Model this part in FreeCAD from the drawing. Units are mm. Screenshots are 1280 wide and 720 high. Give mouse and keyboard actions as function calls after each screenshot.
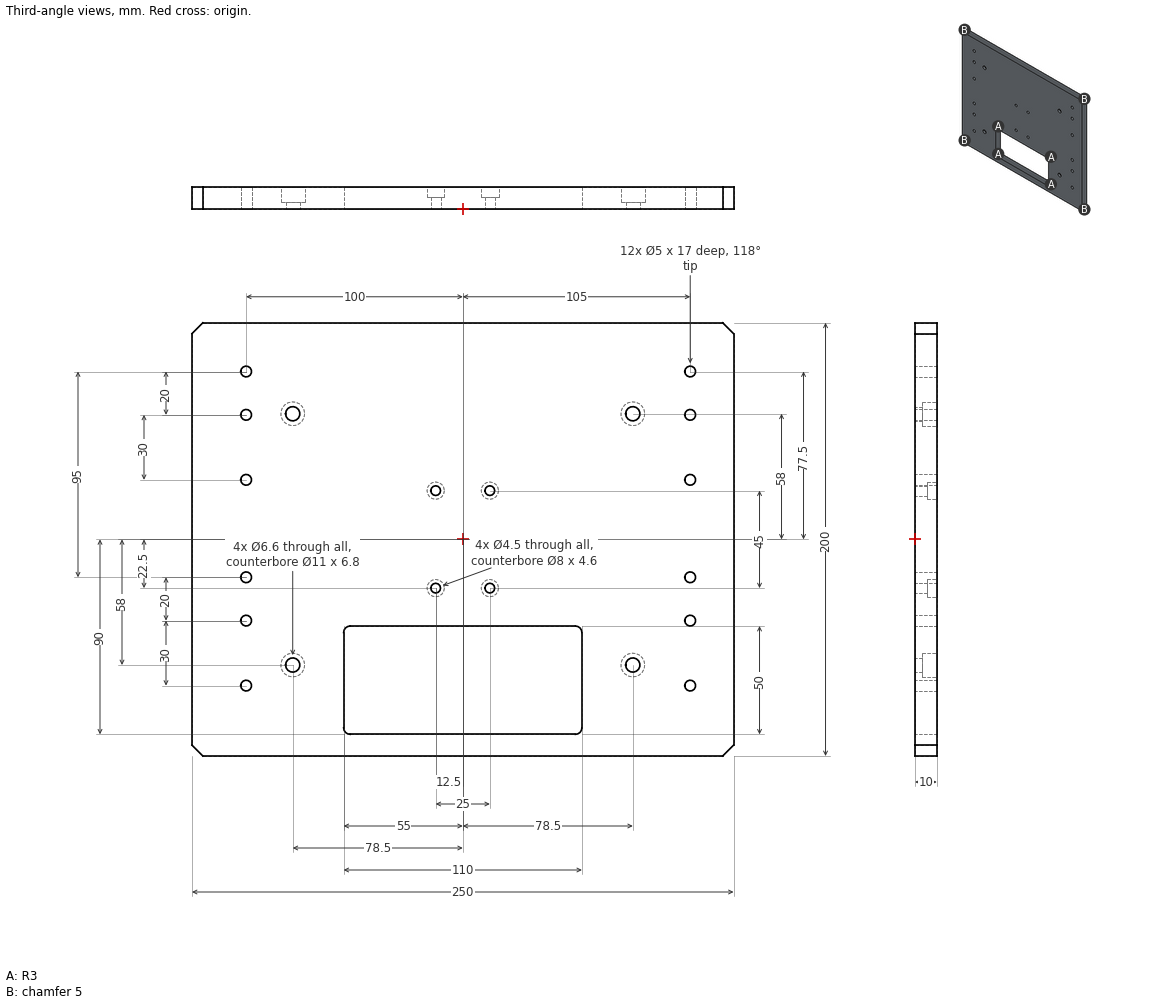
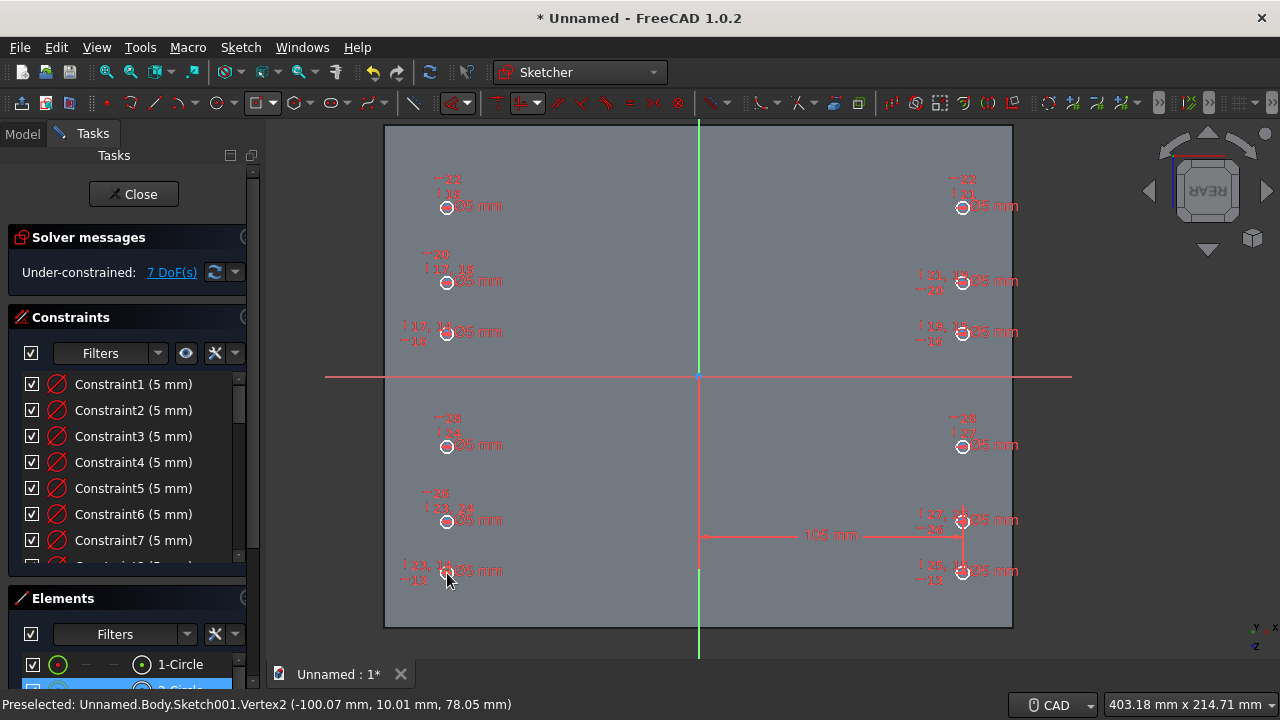
key(l)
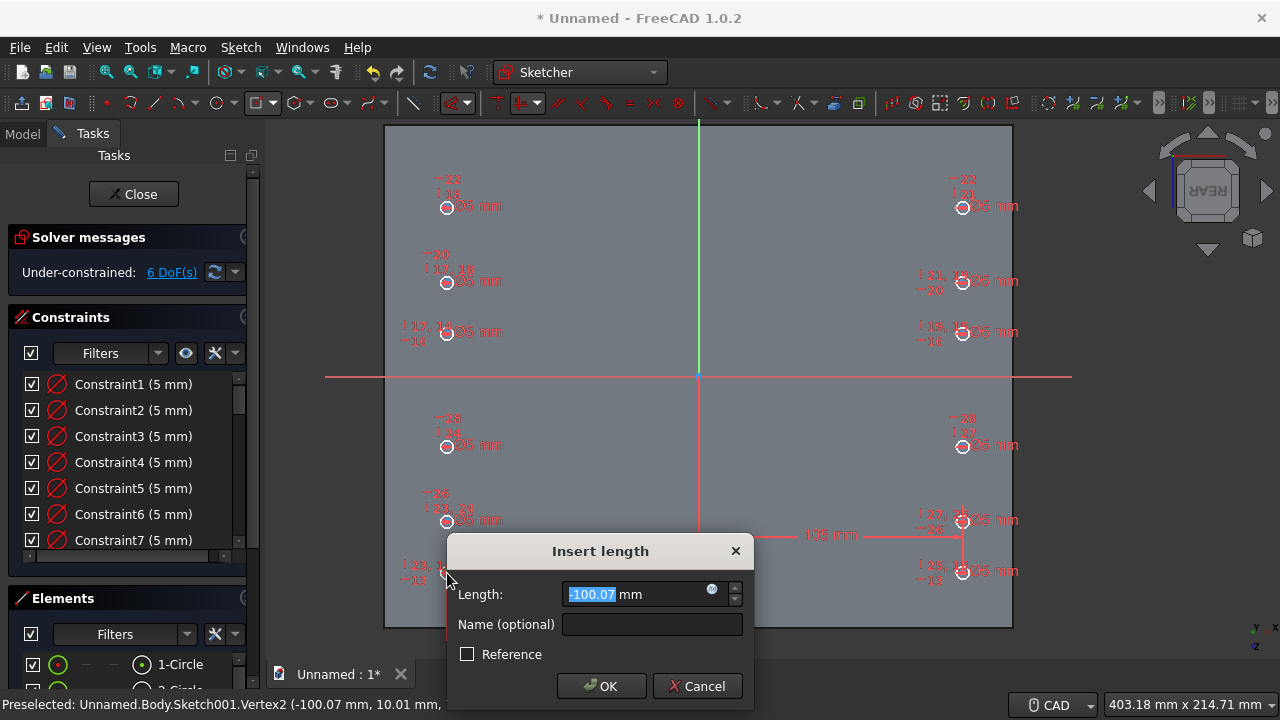
text(-100)
key(Return)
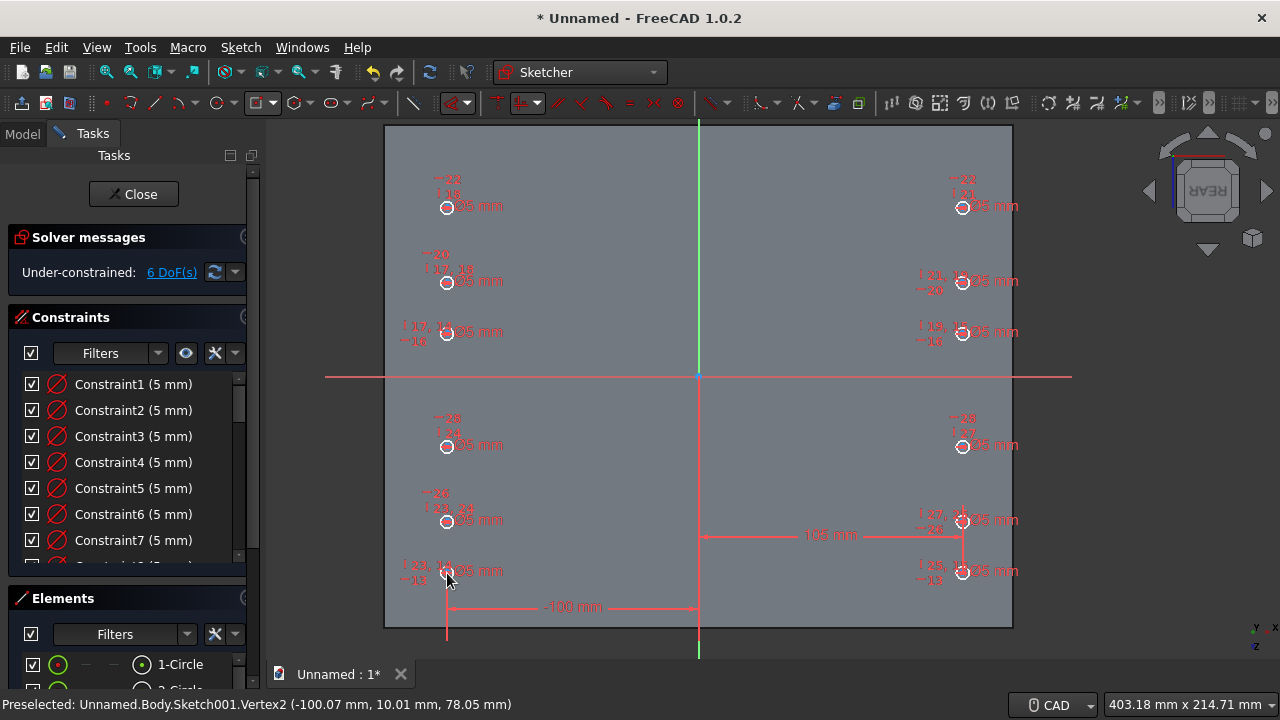
click(447, 573)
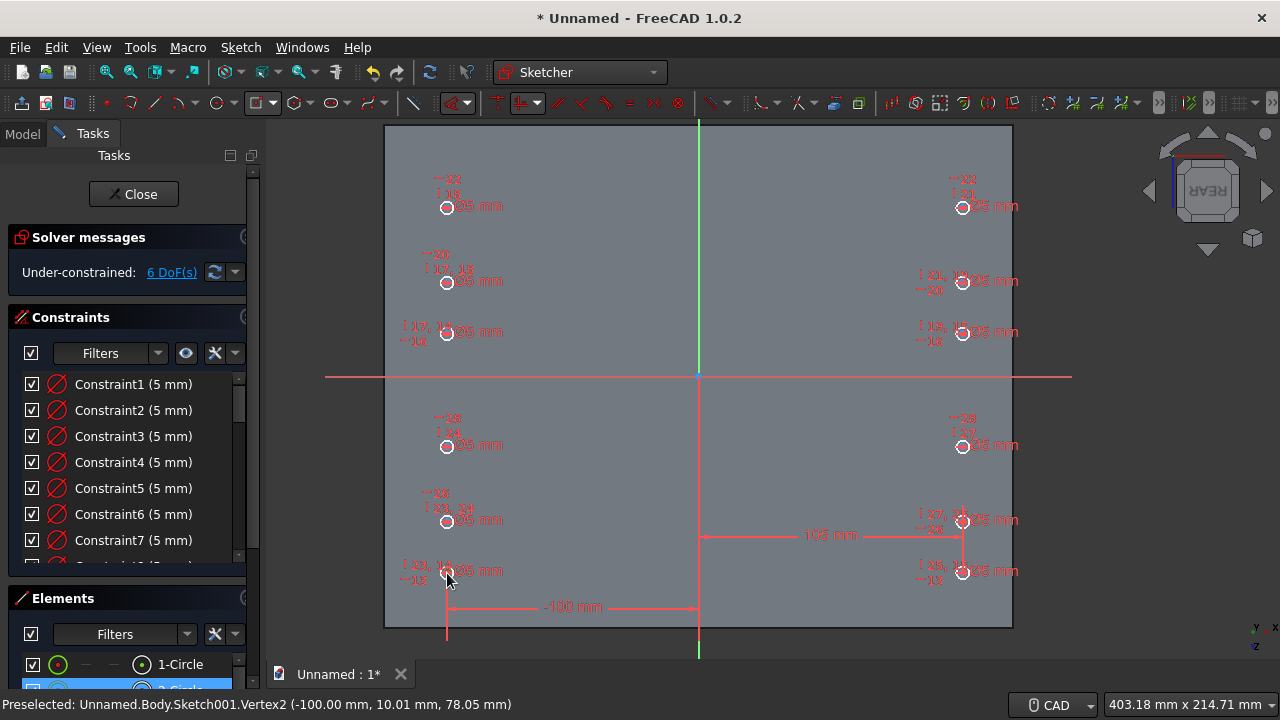
click(447, 334)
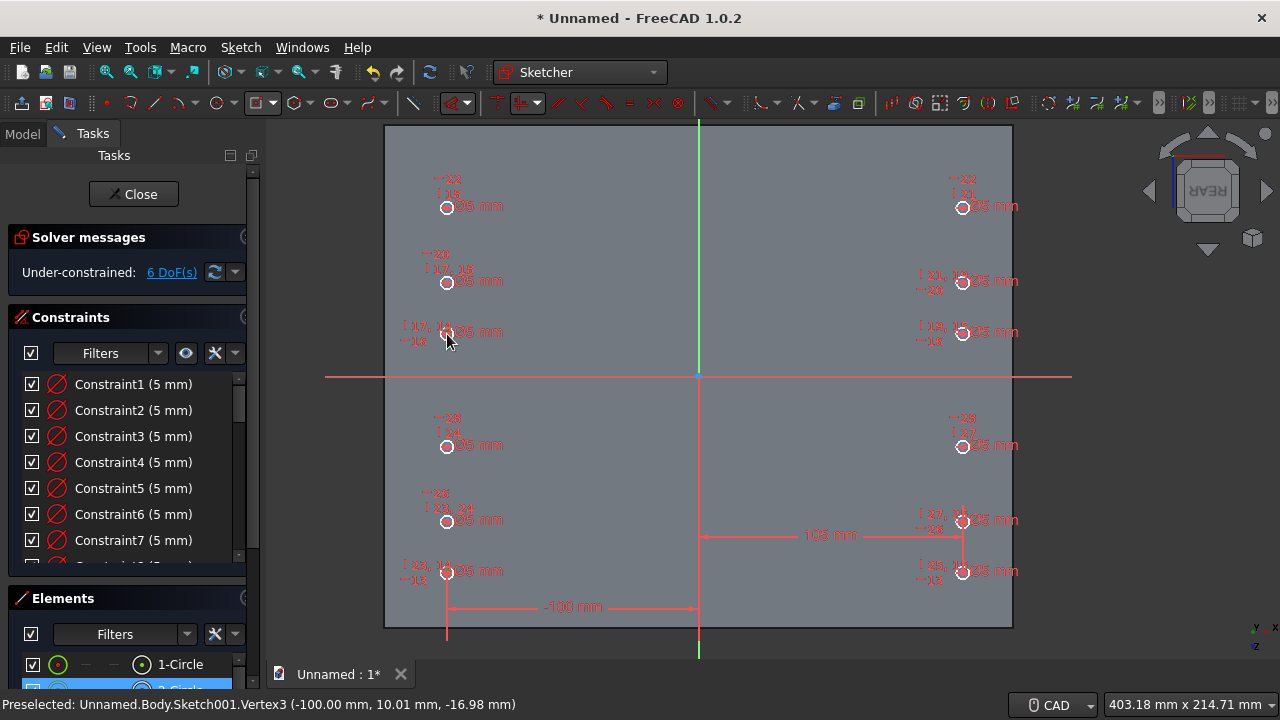
click(470, 104)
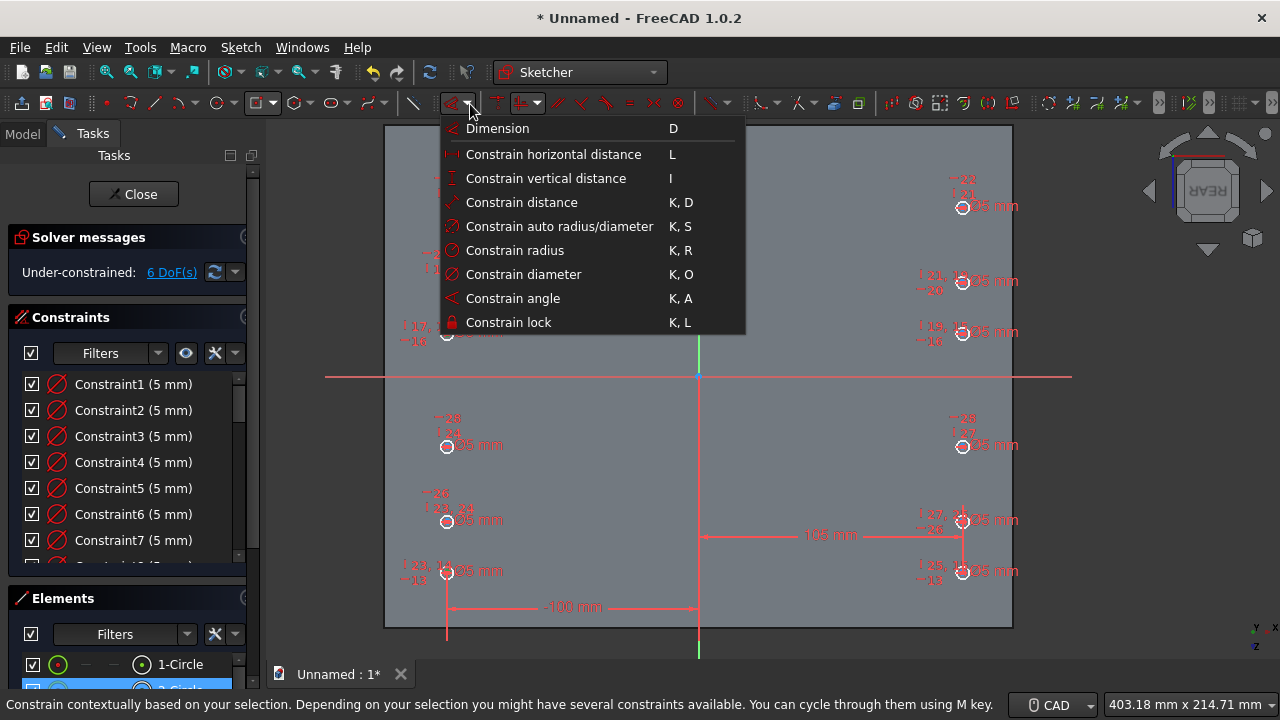
click(593, 178)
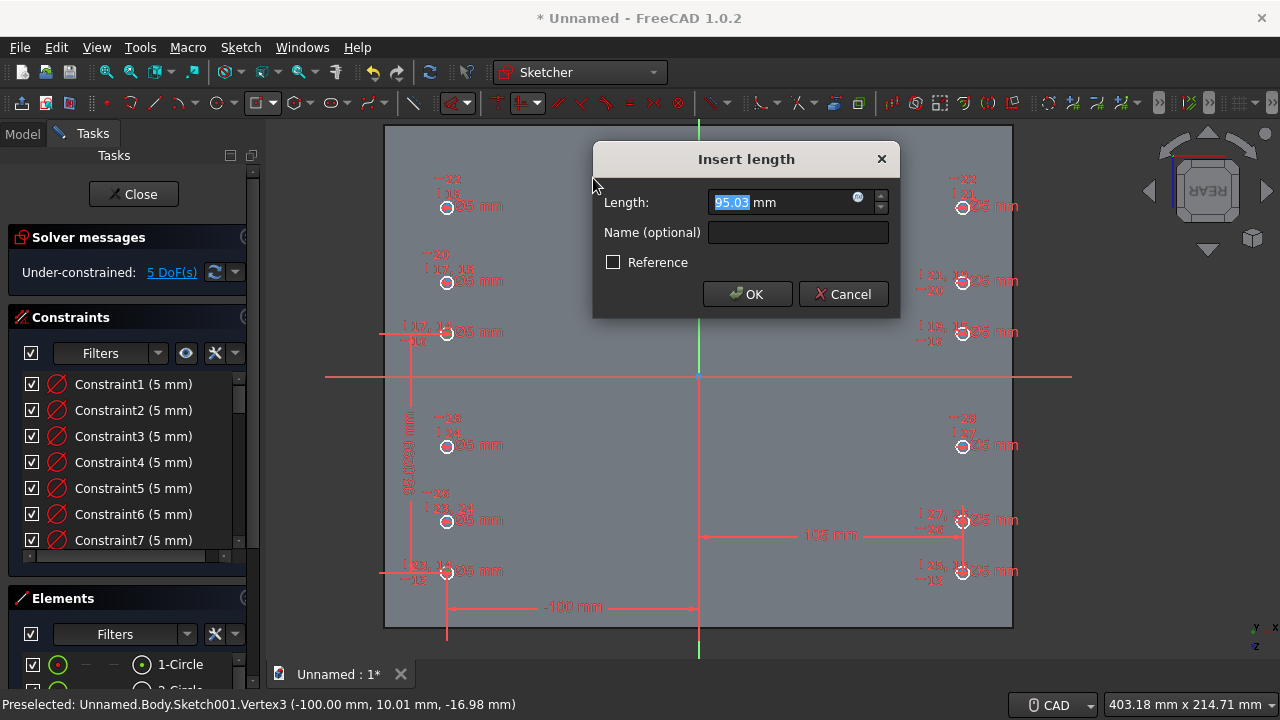
text(95)
key(Return)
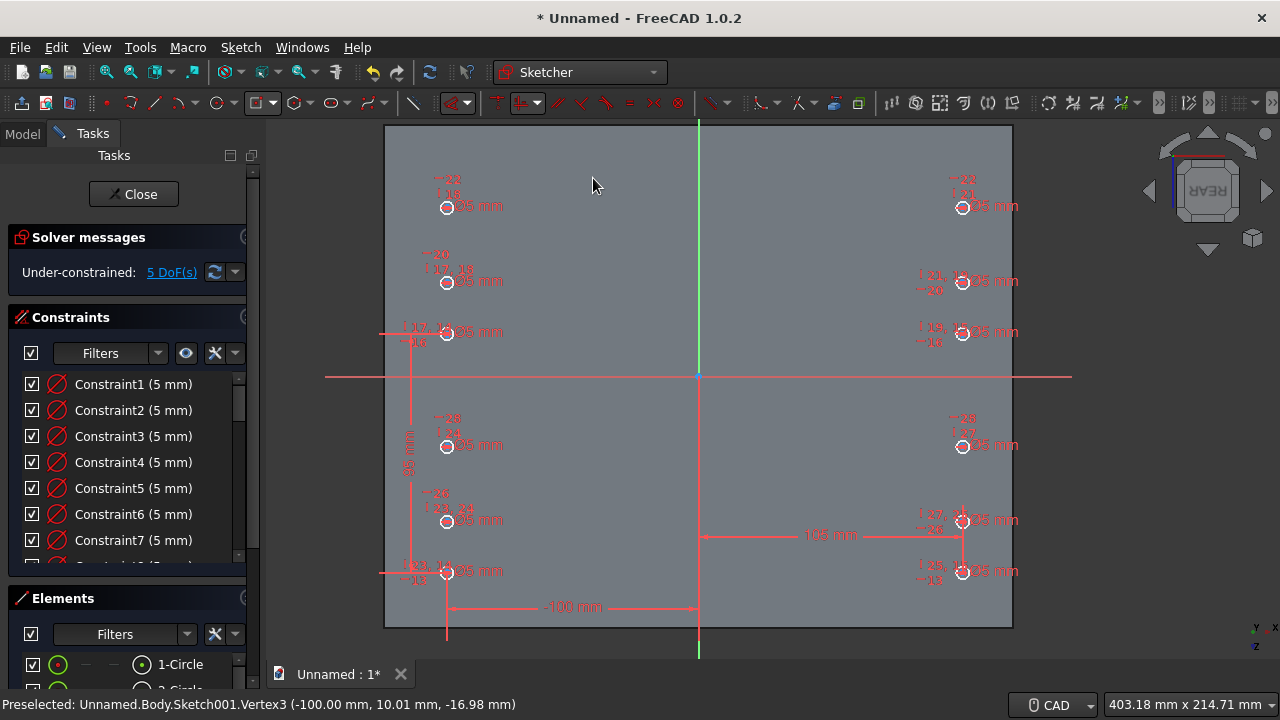
click(447, 334)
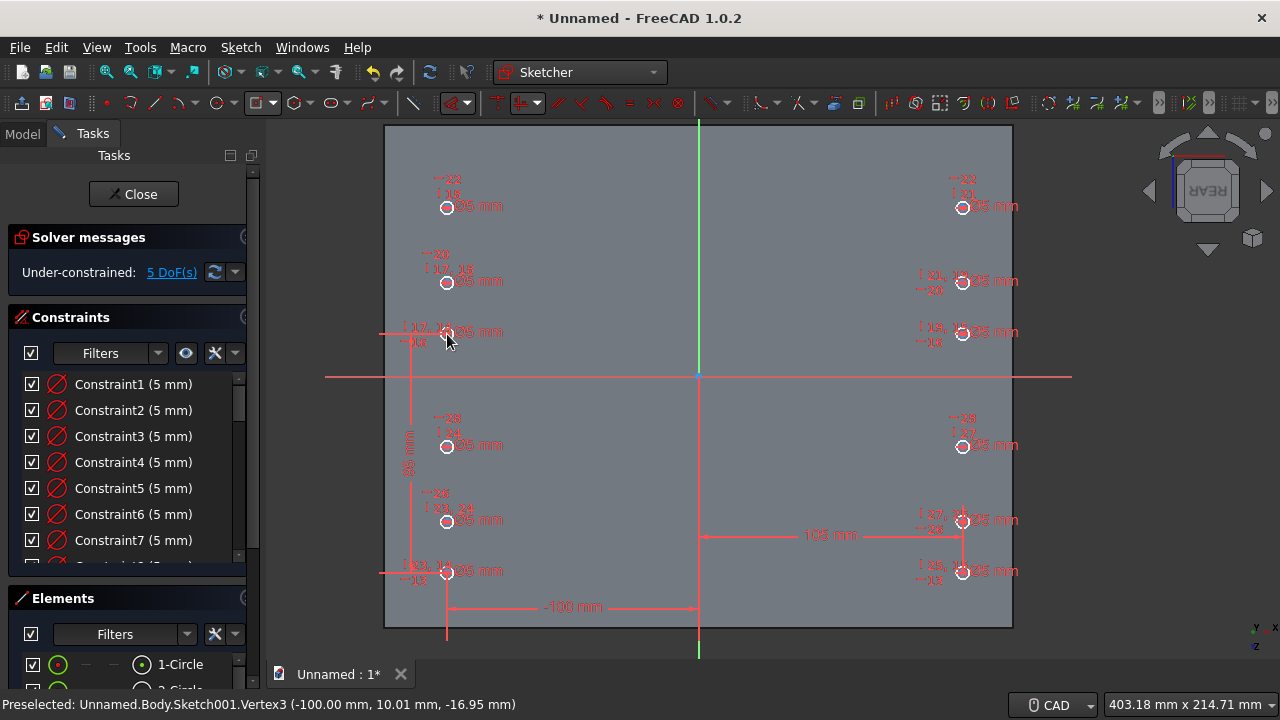
click(447, 283)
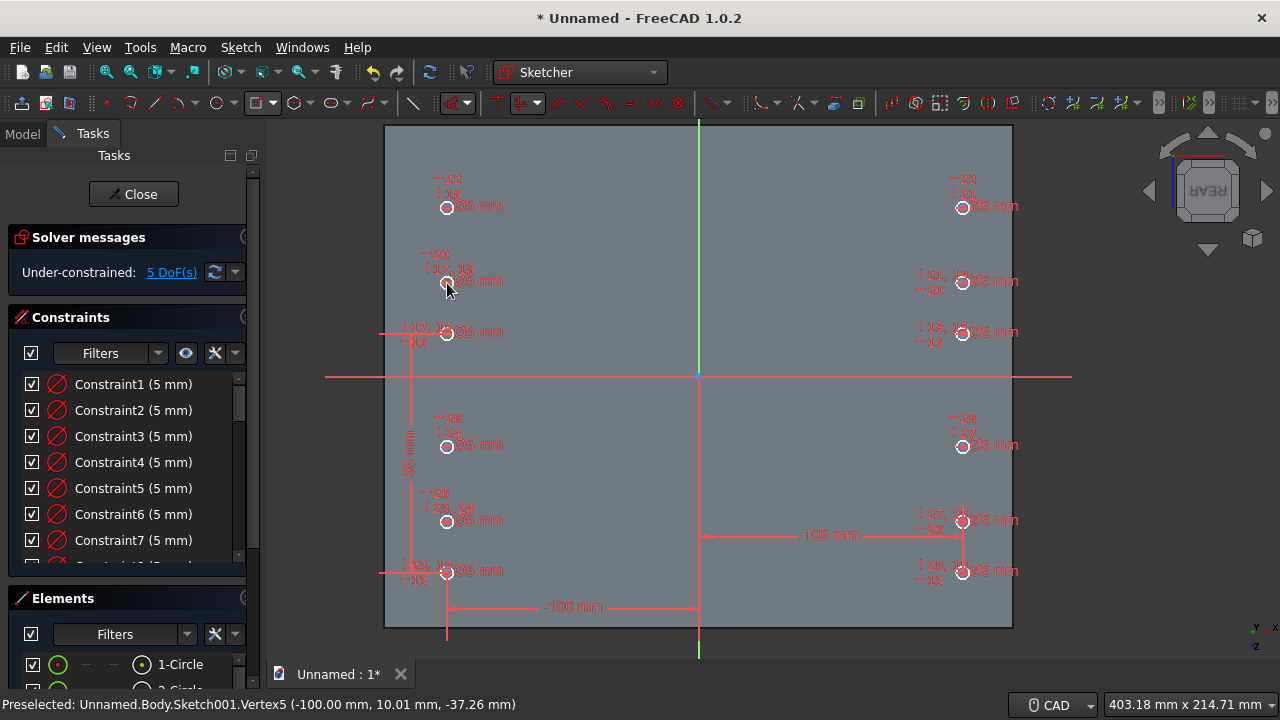
key(i)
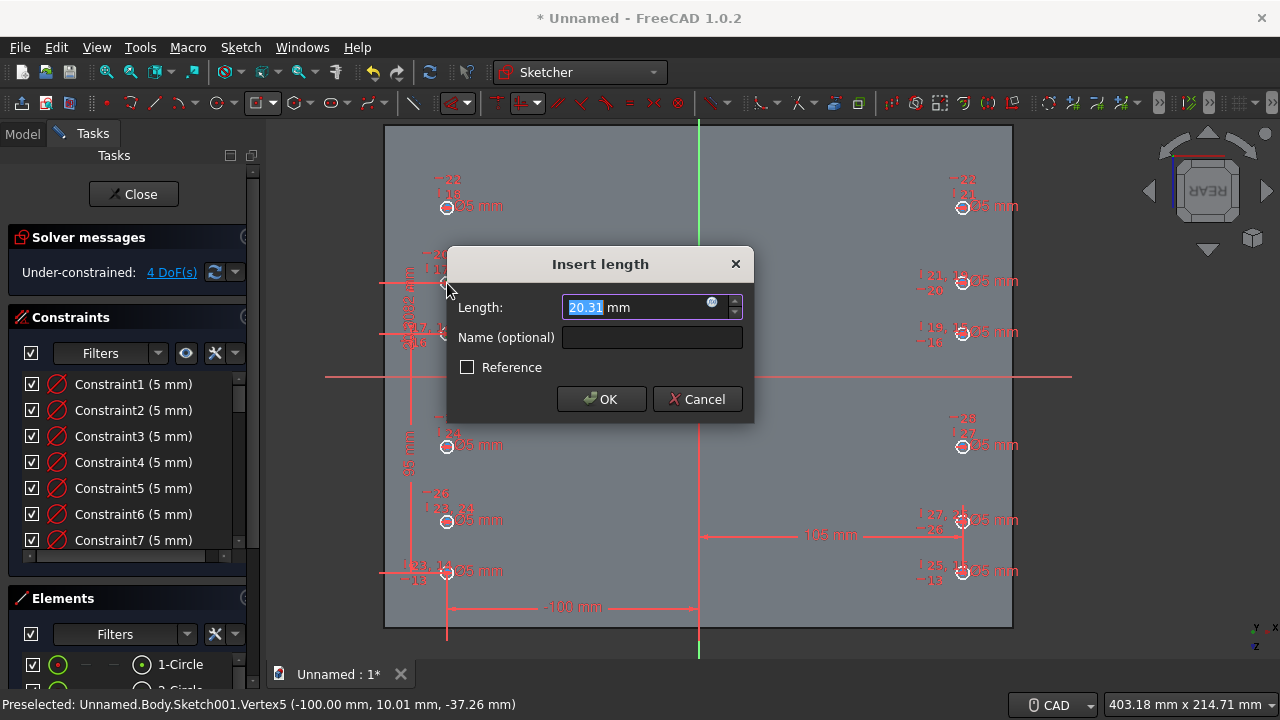
text(20)
key(Return)